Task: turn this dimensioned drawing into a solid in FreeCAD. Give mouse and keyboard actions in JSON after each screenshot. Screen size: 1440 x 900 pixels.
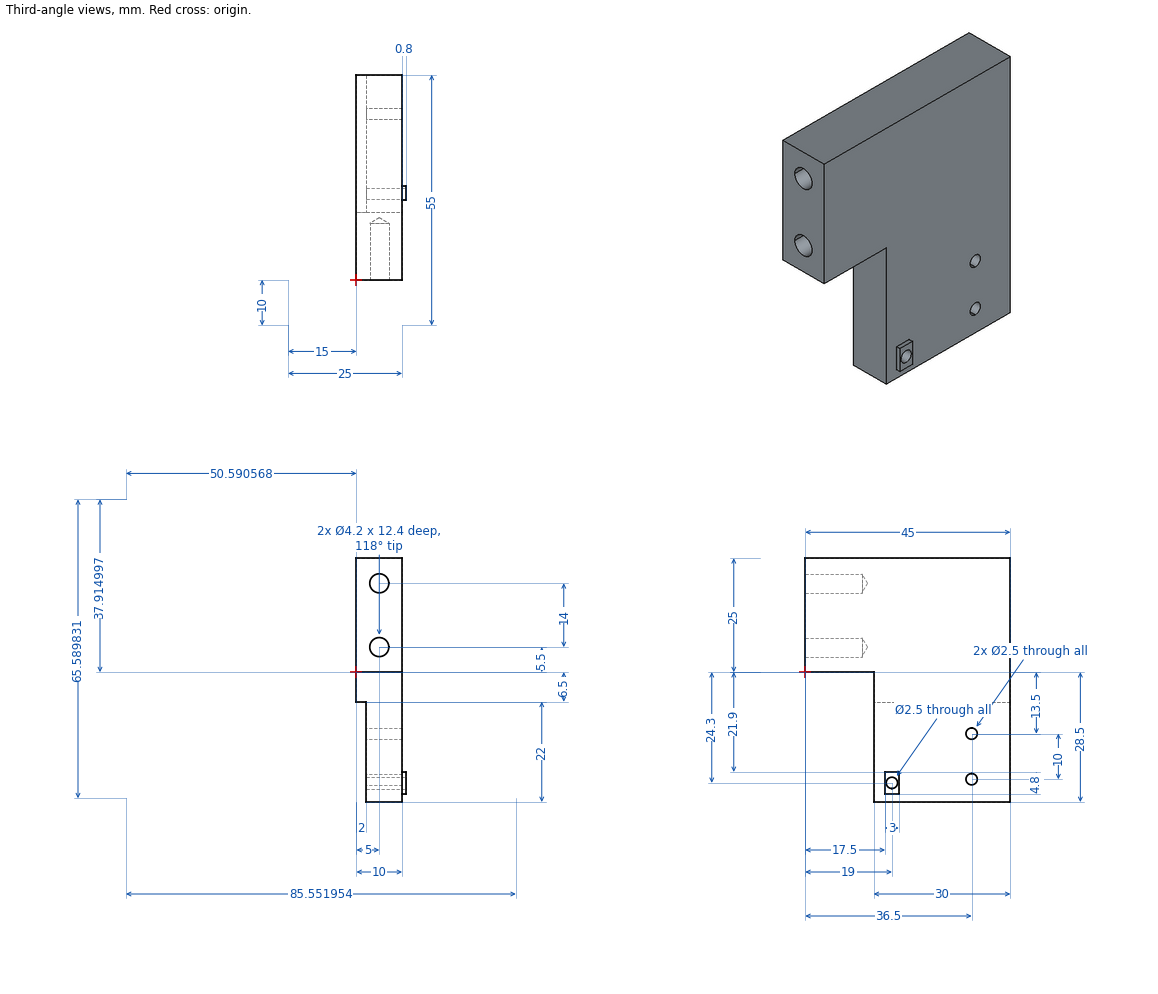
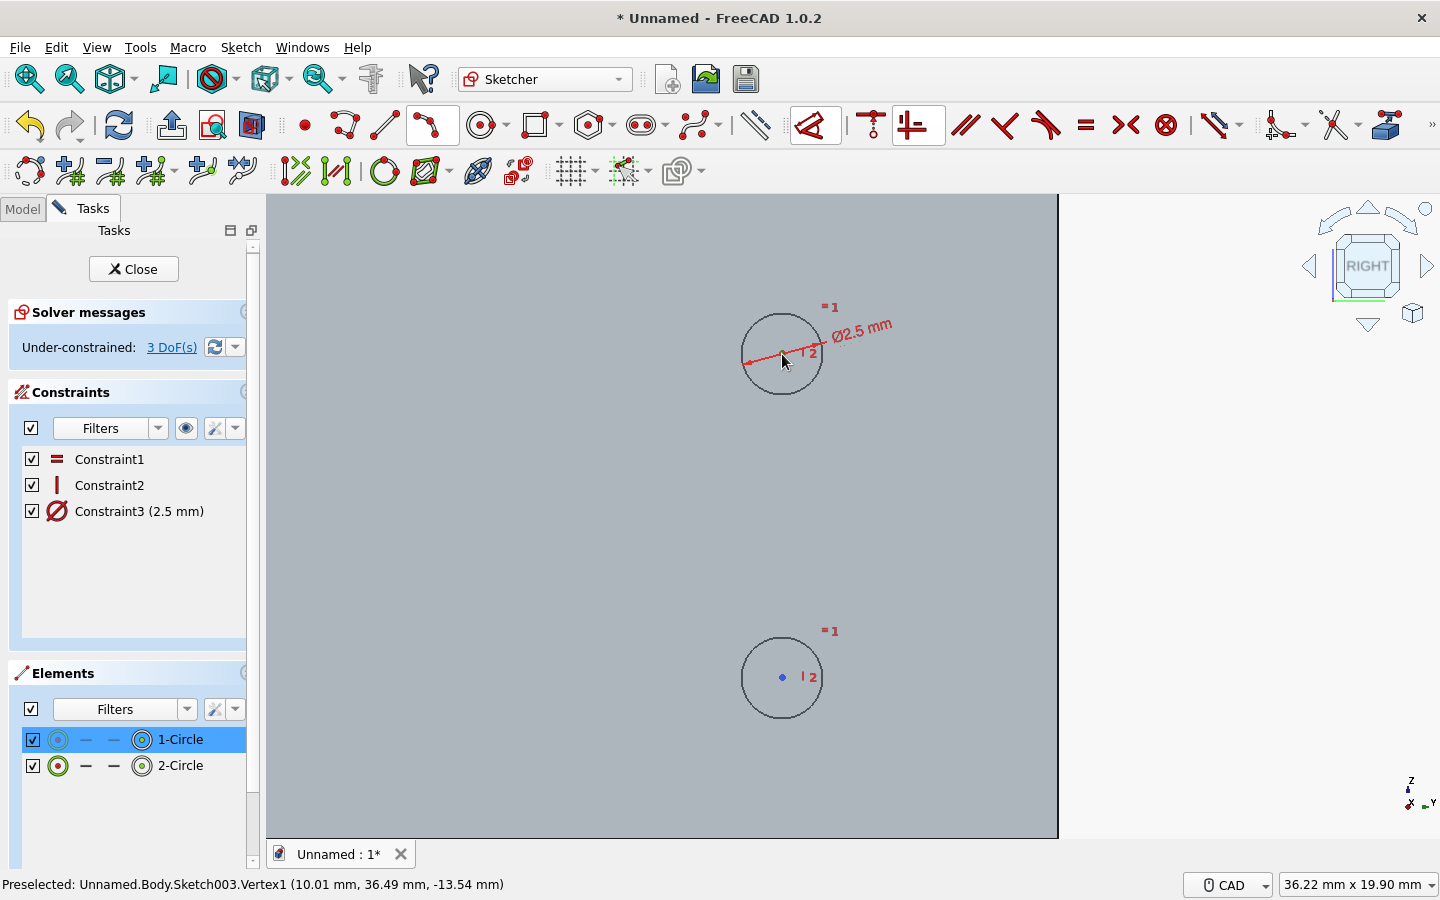
{"action": "left_click", "coordinate": [782, 678]}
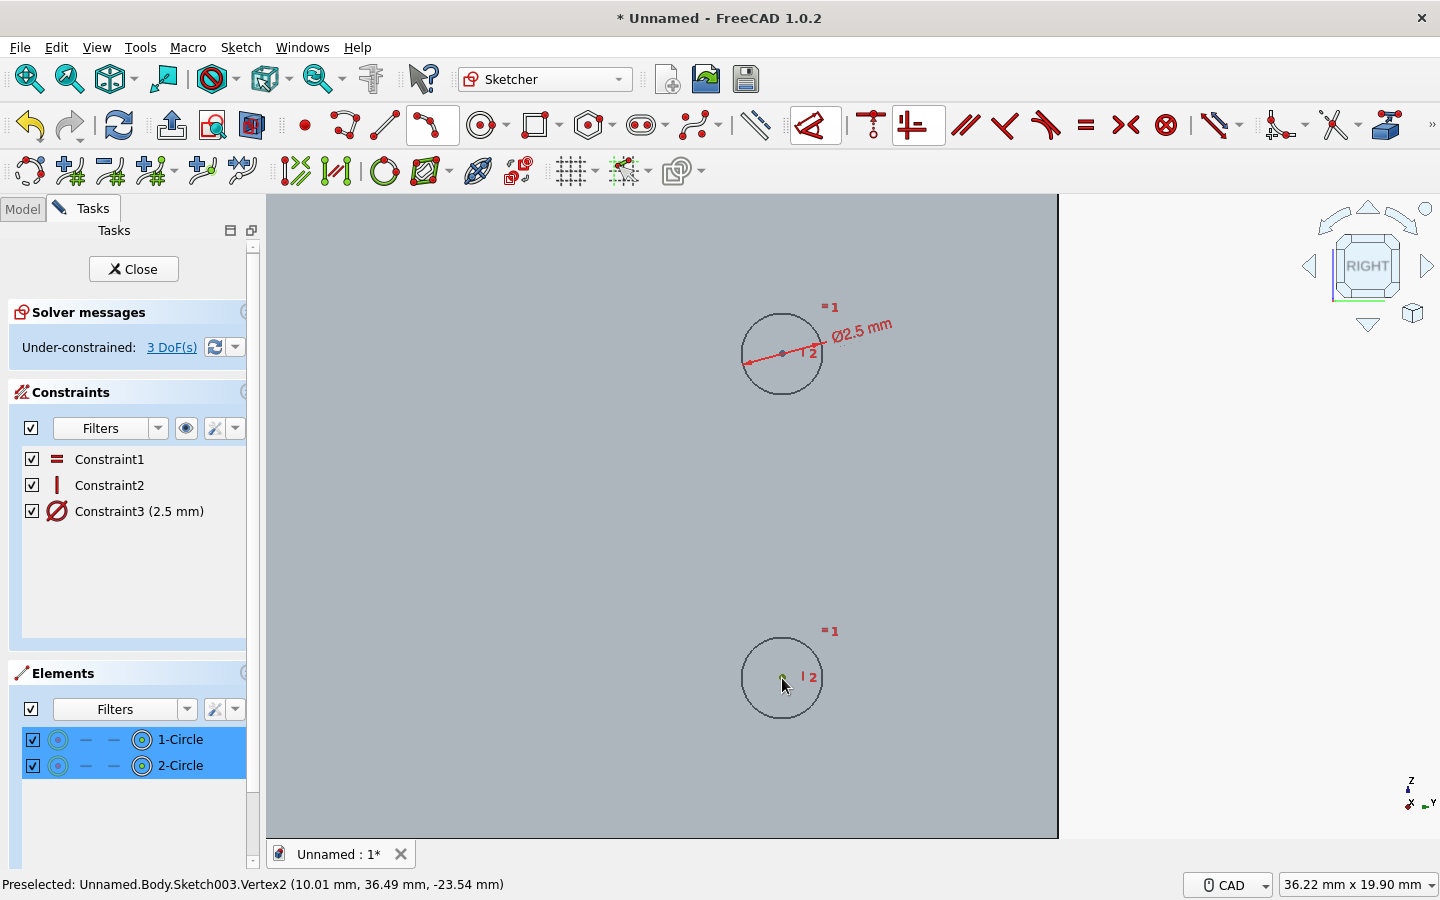
{"action": "left_click", "coordinate": [836, 126]}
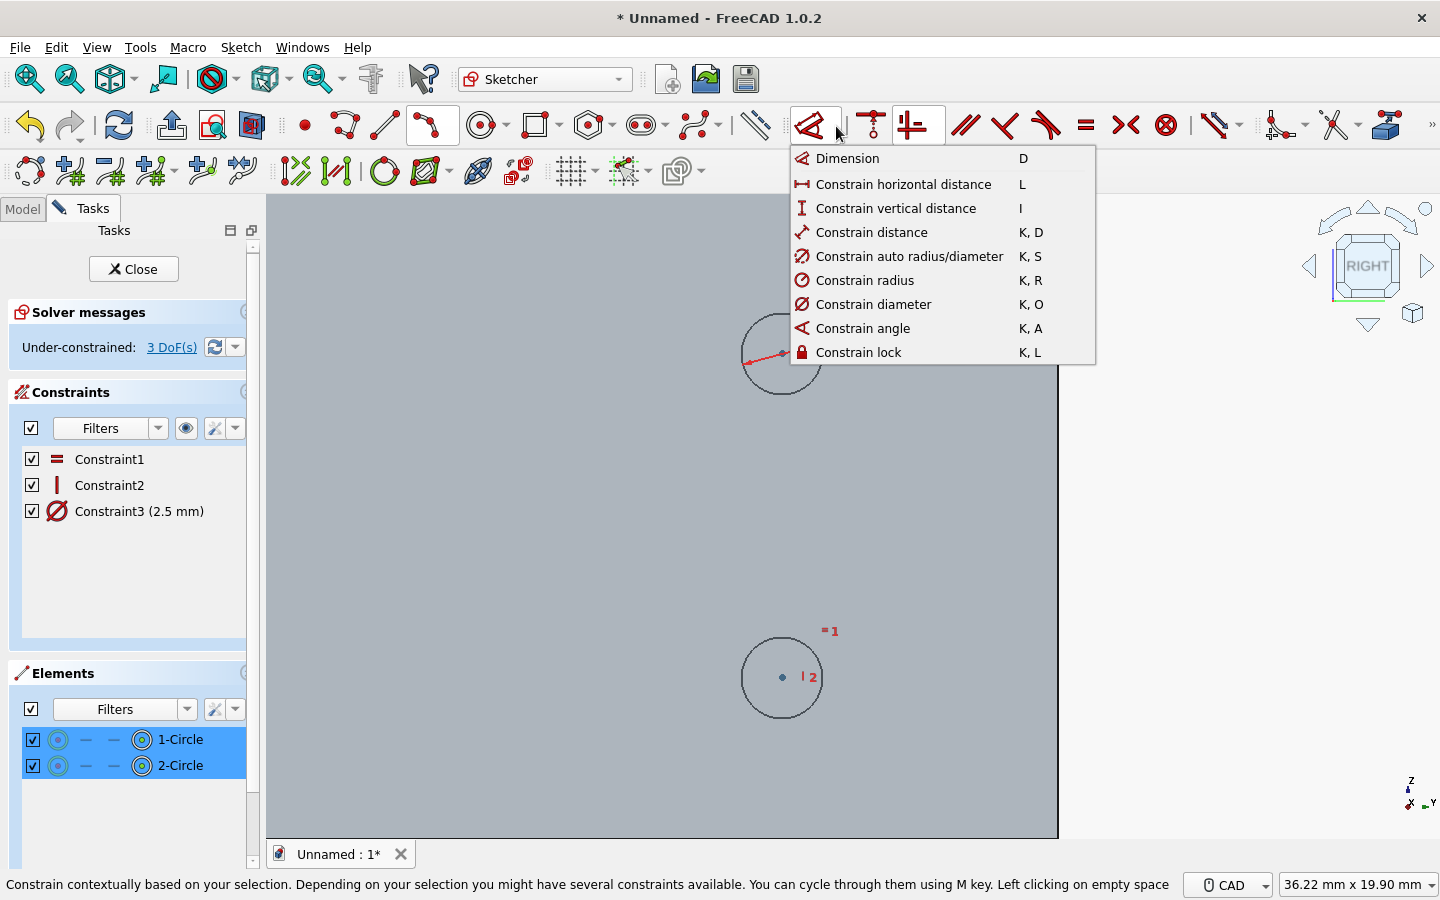
{"action": "left_click", "coordinate": [943, 208]}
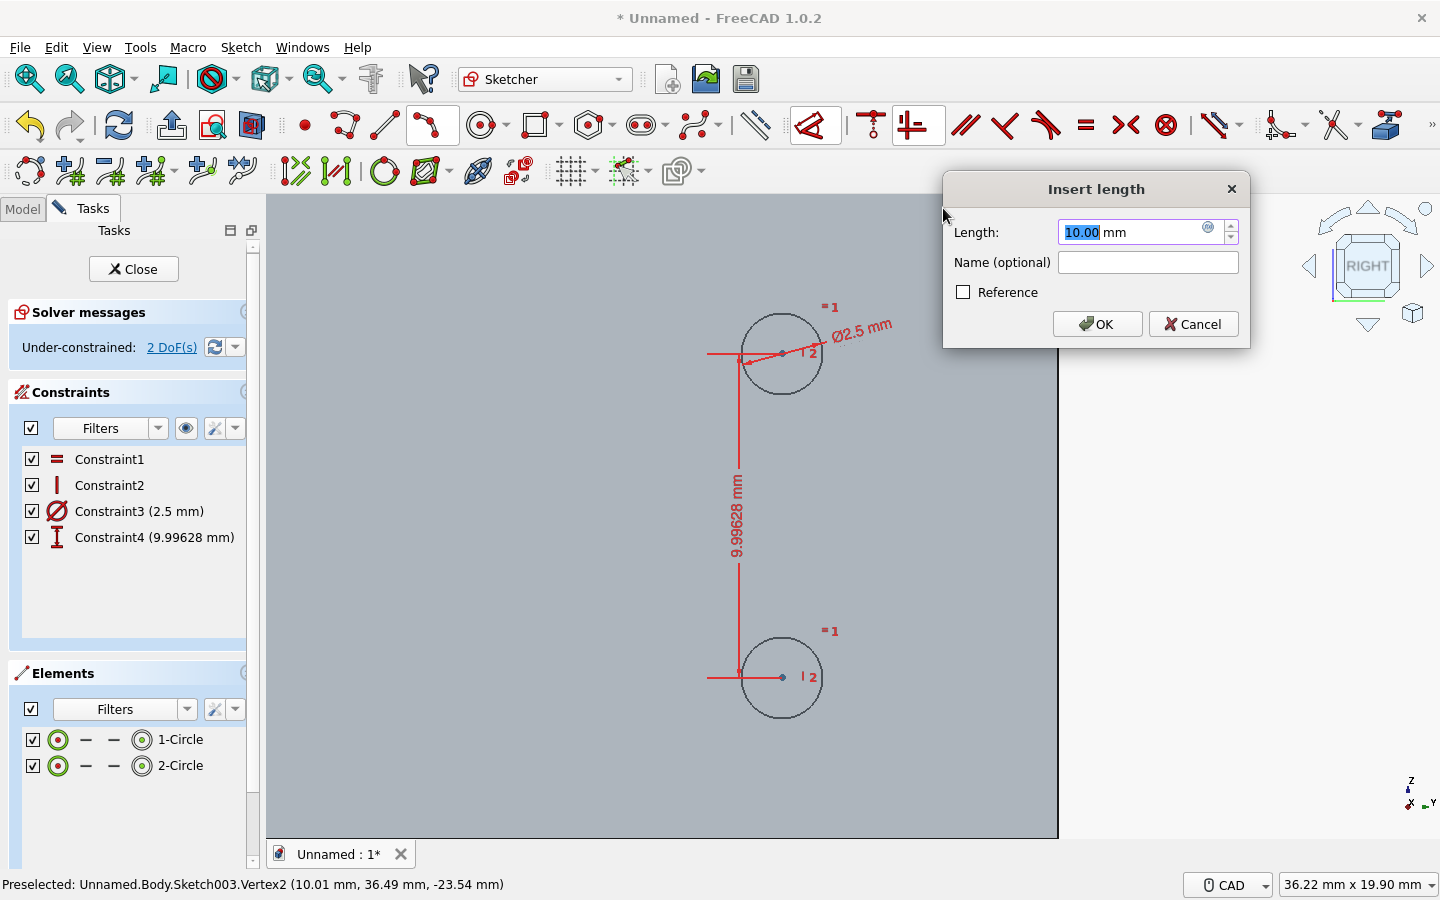
{"action": "type", "text": "10"}
{"action": "key", "text": "Return"}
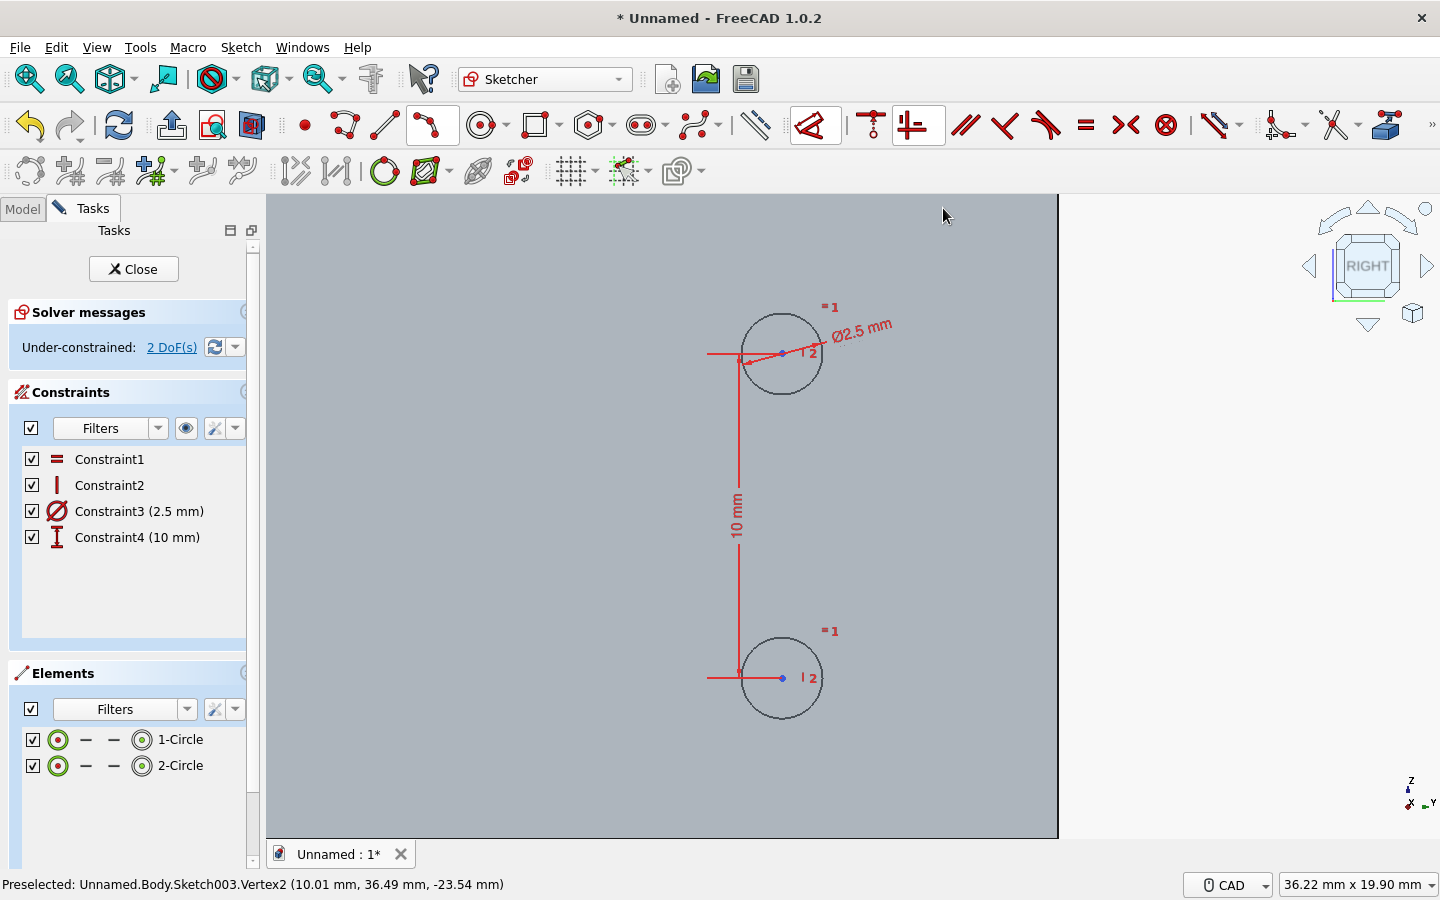
{"action": "left_click", "coordinate": [782, 354]}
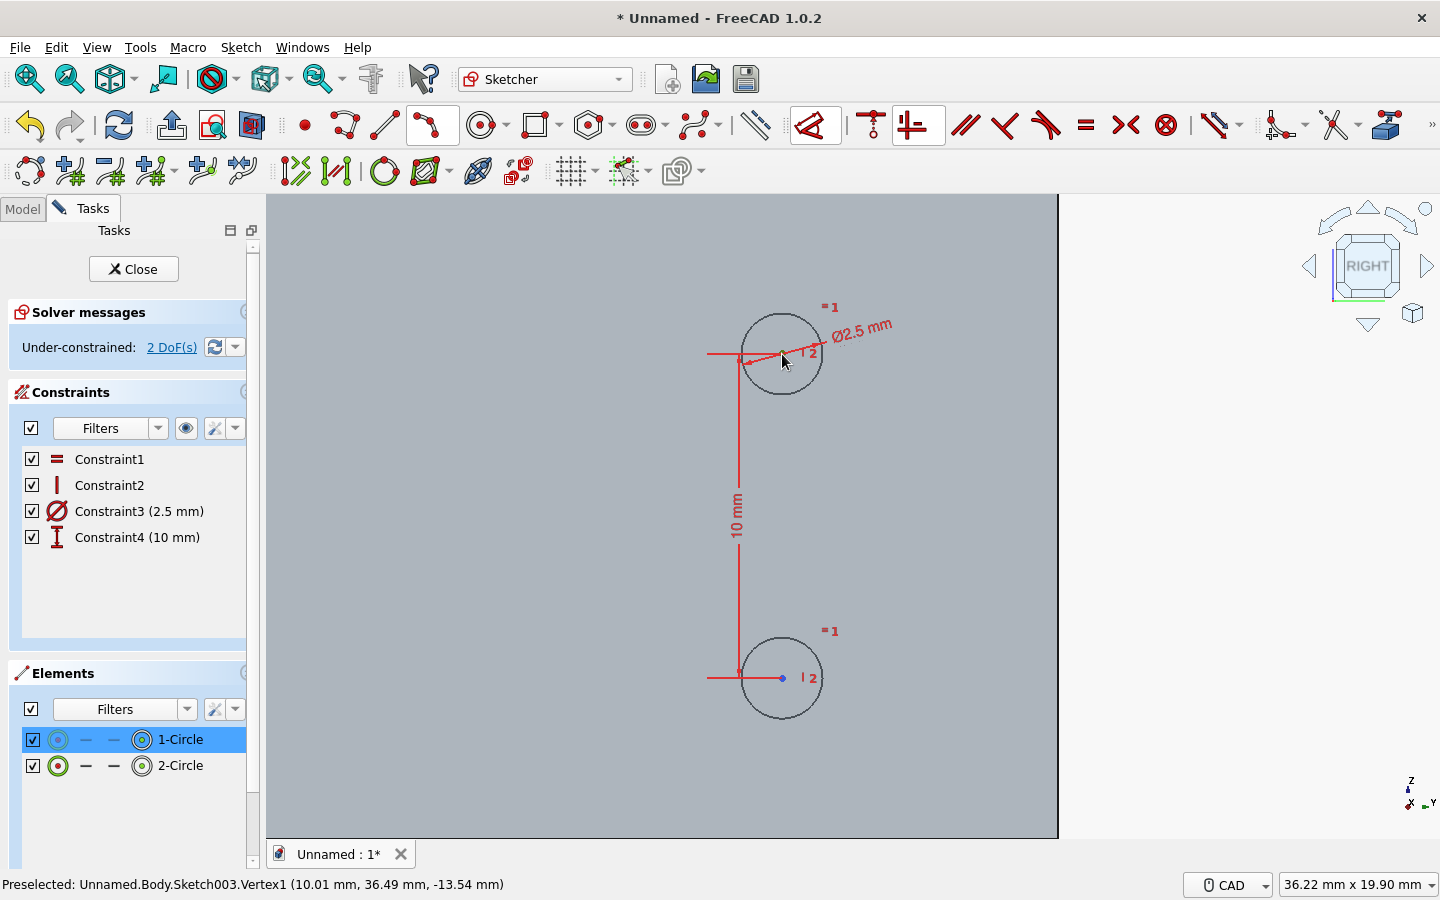
{"action": "key", "text": "l"}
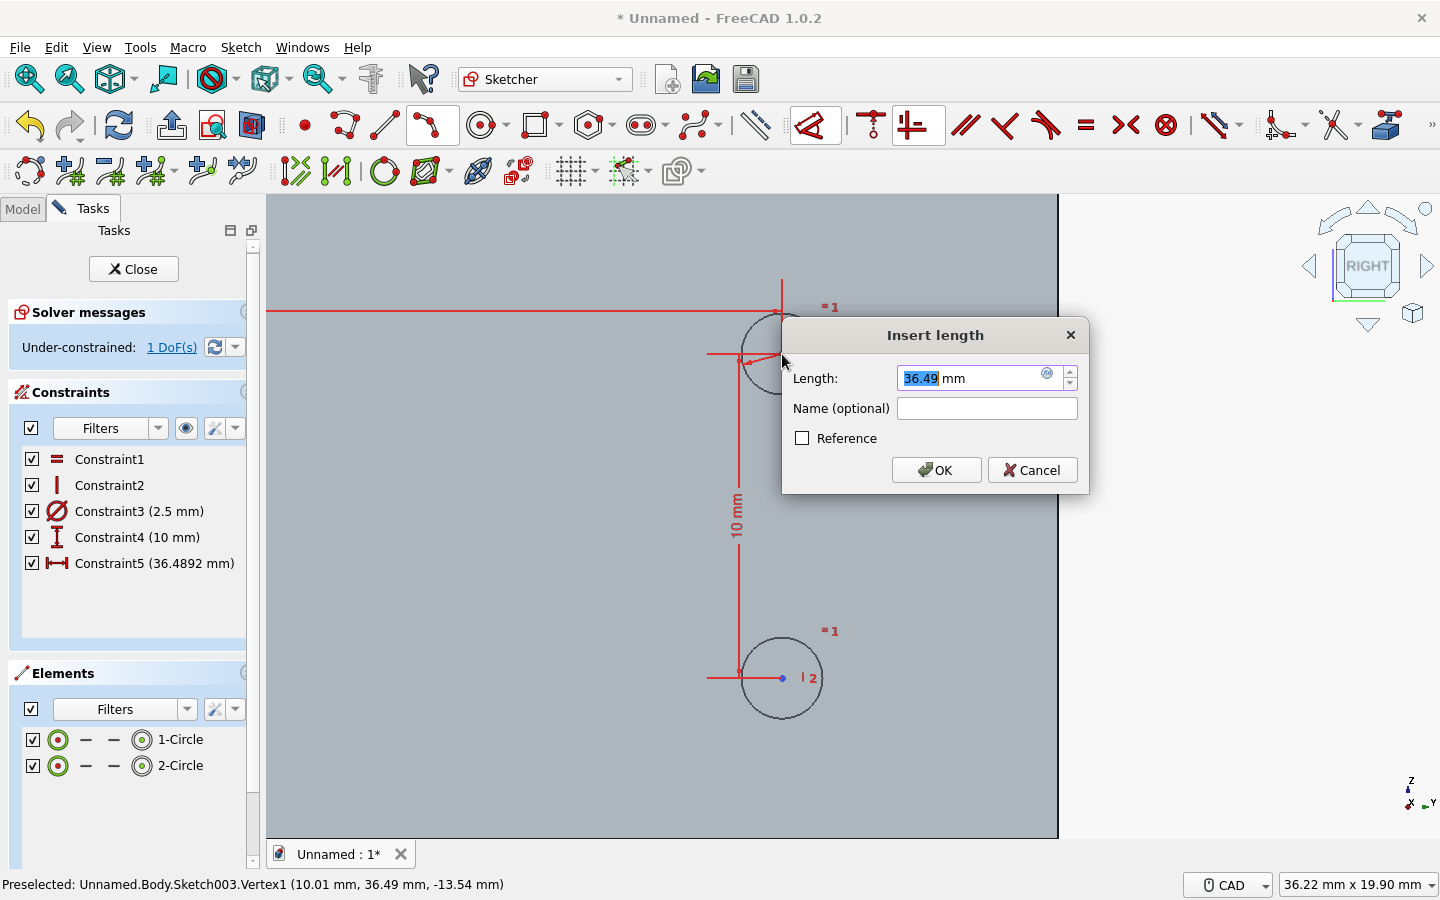
{"action": "type", "text": "36.5"}
{"action": "key", "text": "Return"}